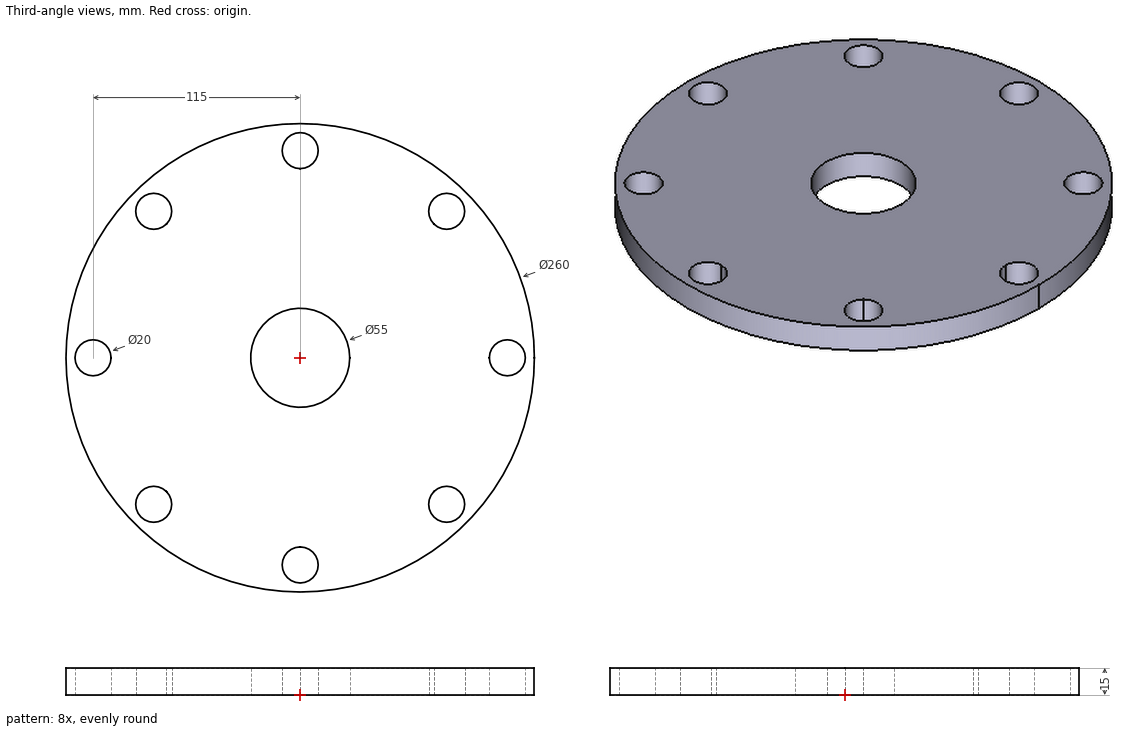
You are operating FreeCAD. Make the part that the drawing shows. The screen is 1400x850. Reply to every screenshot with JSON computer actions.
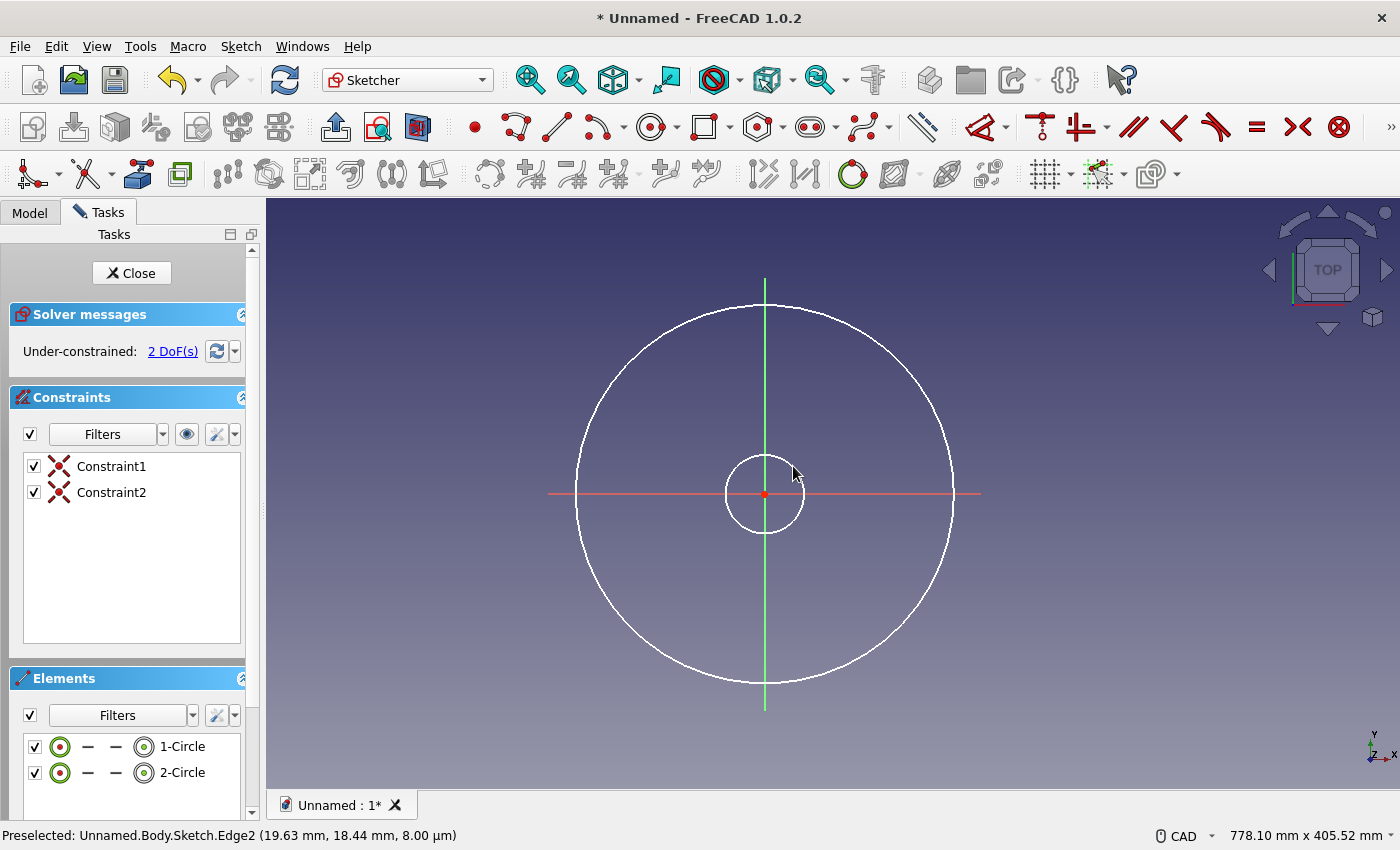
{"action": "left_click", "coordinate": [980, 128]}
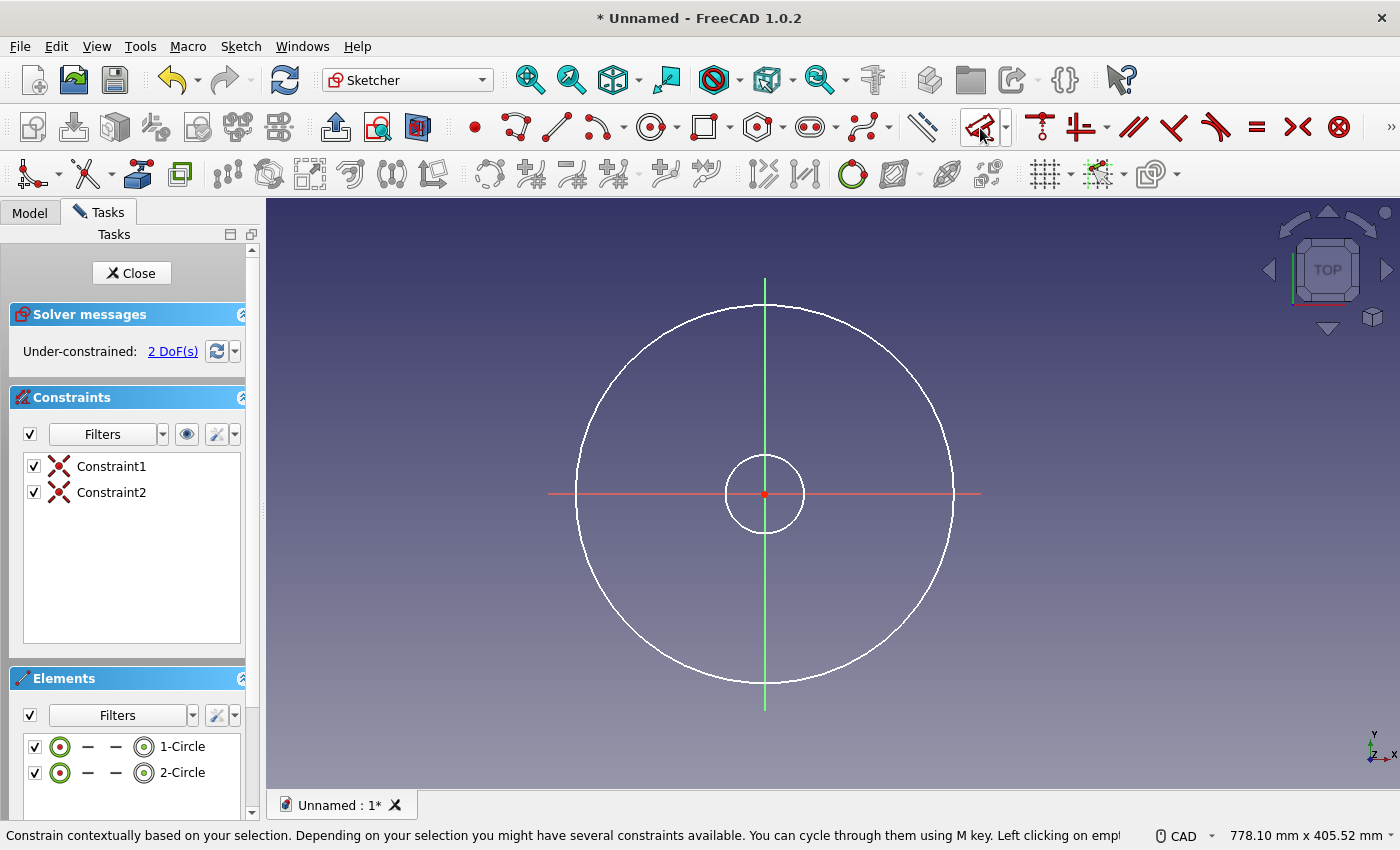
{"action": "left_click", "coordinate": [898, 360]}
{"action": "left_click", "coordinate": [921, 337]}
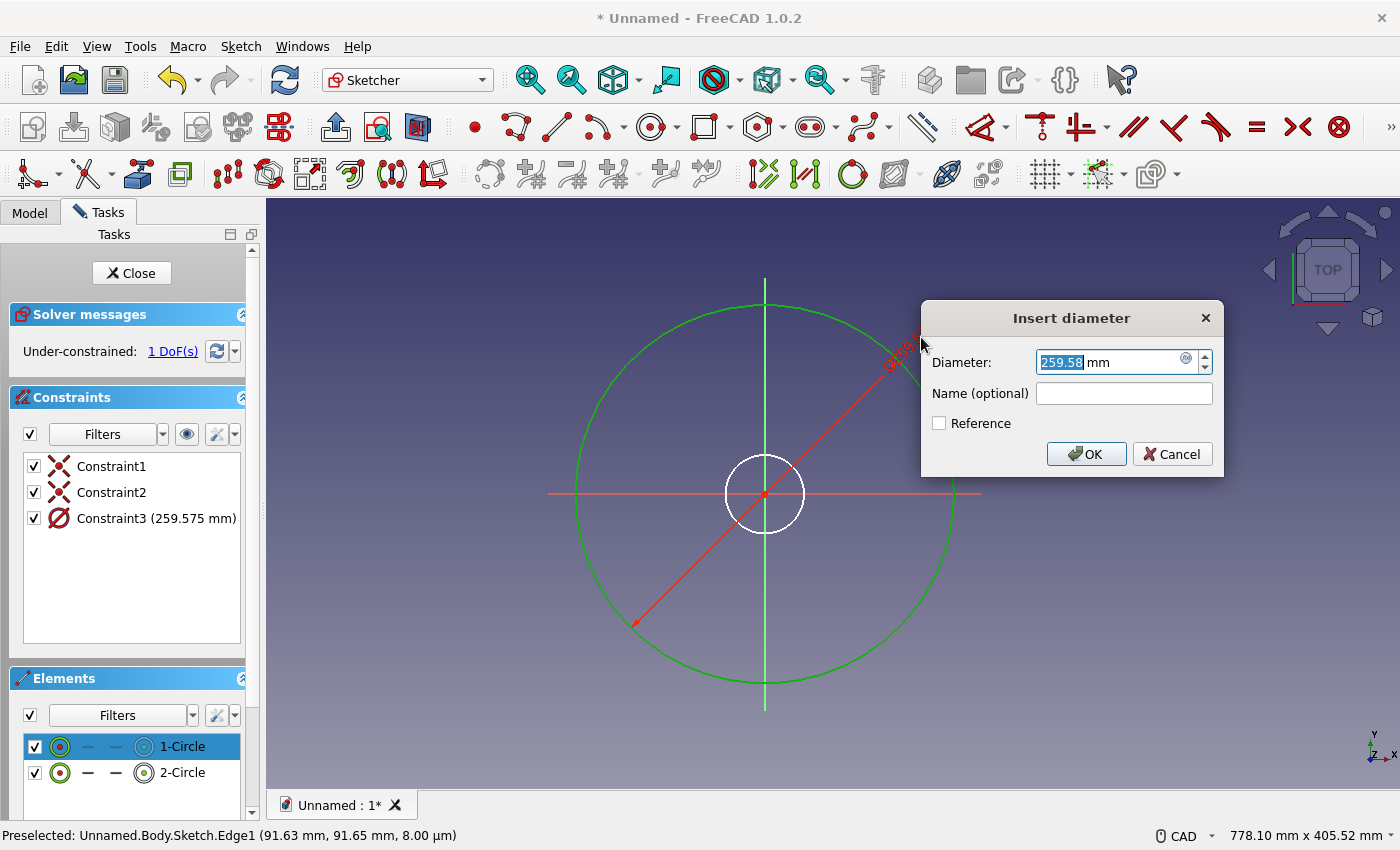
{"action": "type", "text": "260"}
{"action": "key", "text": "Return"}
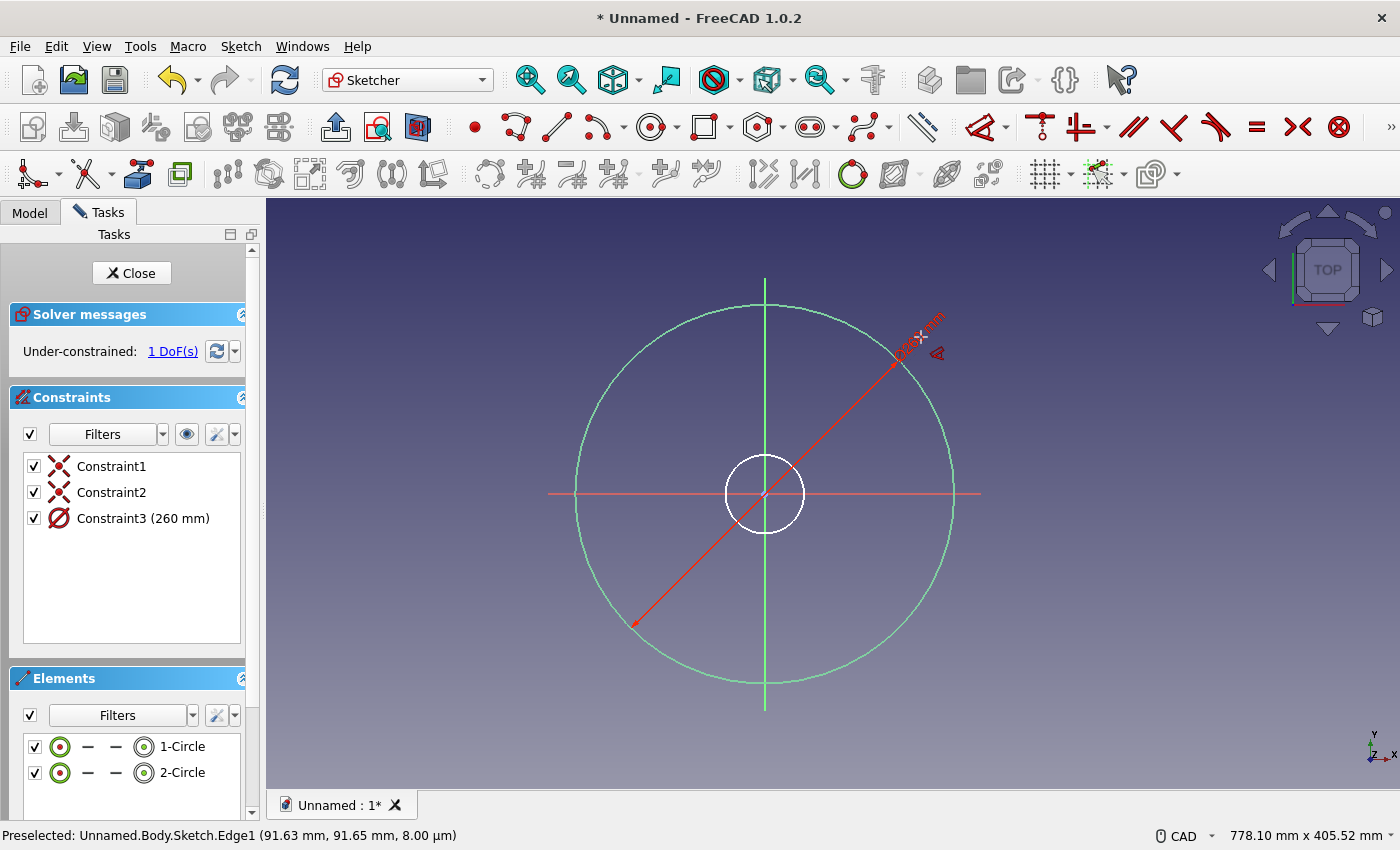
{"action": "left_click", "coordinate": [792, 466]}
{"action": "left_click", "coordinate": [814, 443]}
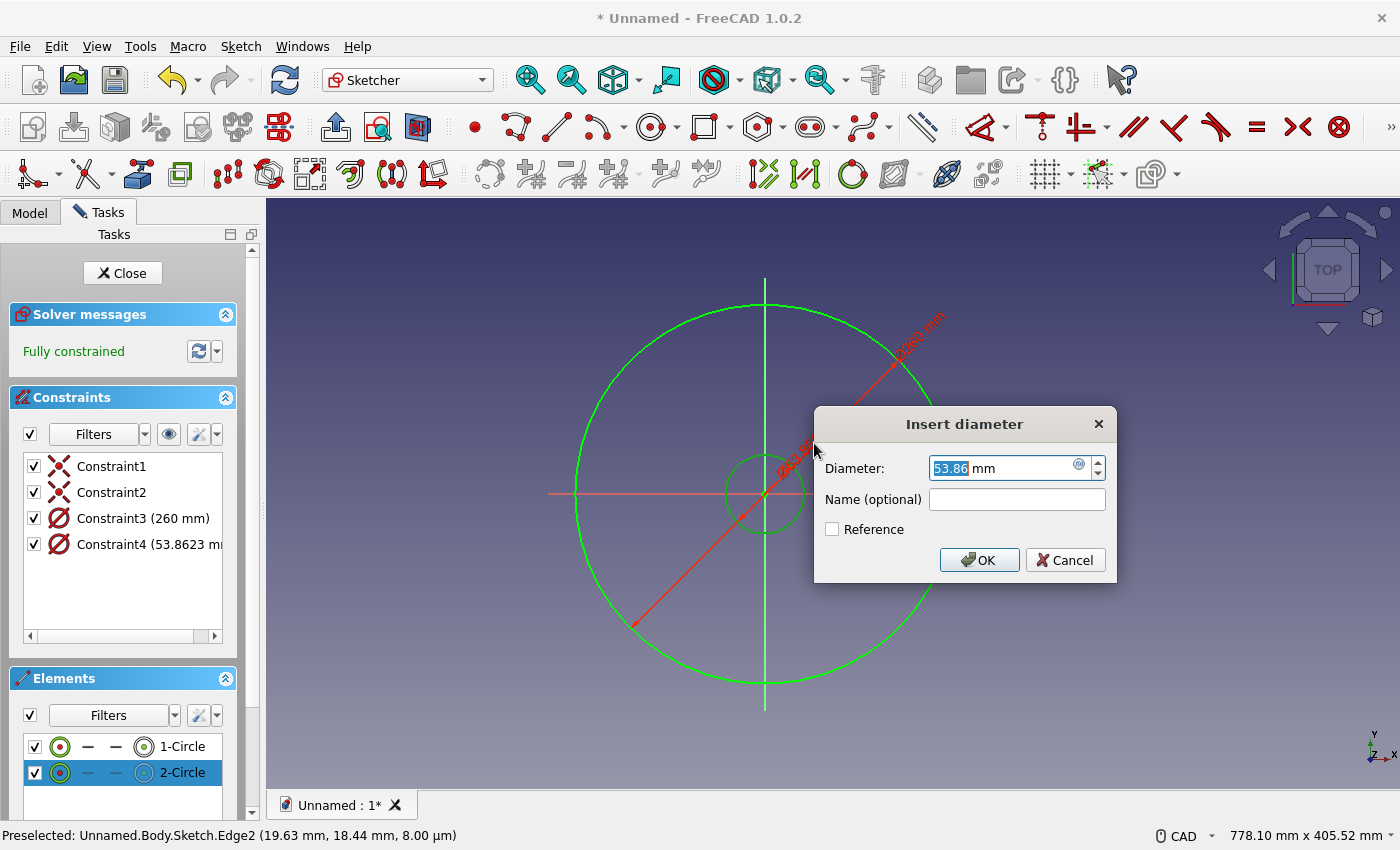
{"action": "type", "text": "55"}
{"action": "key", "text": "Return"}
{"action": "key", "text": "Escape"}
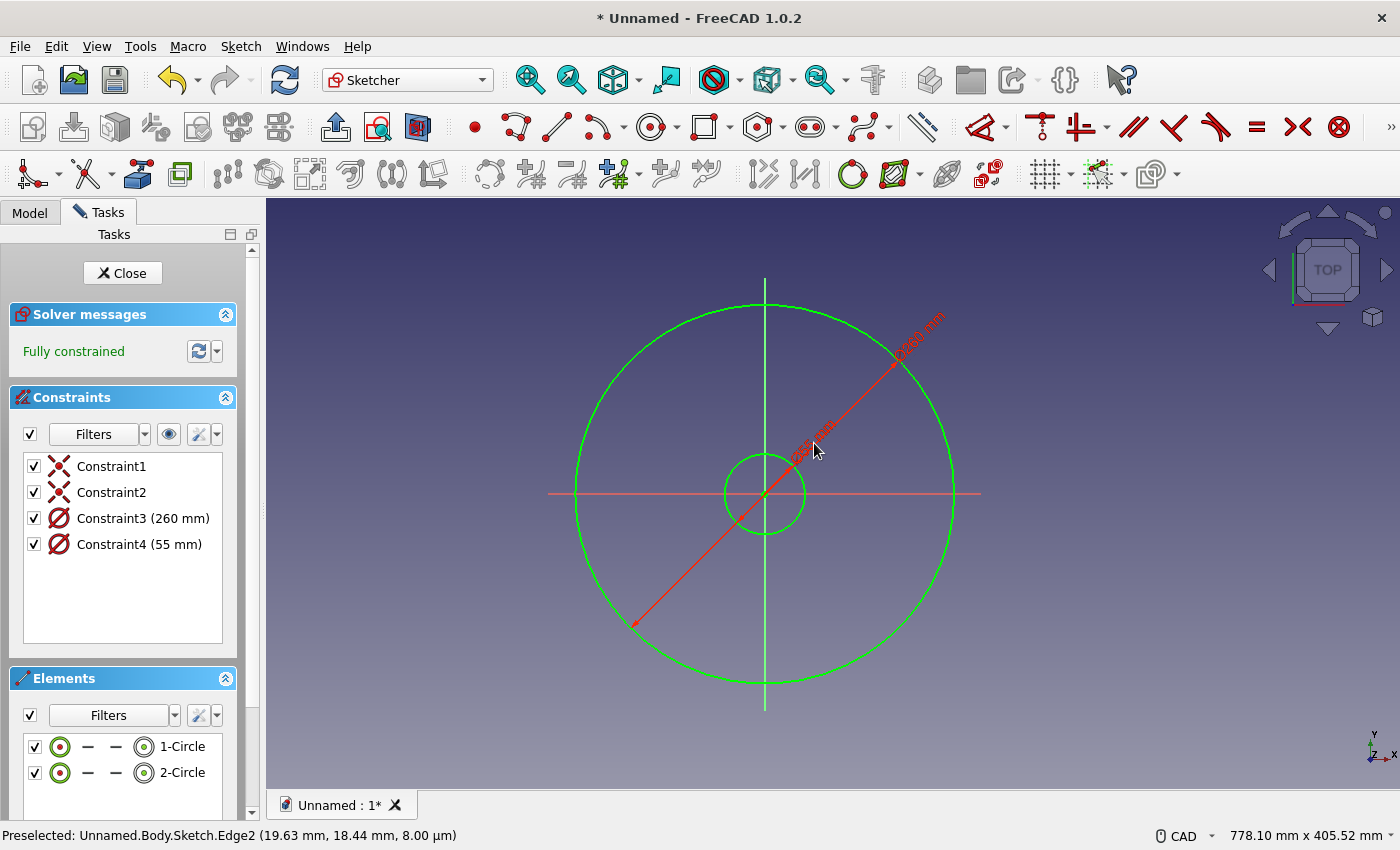
{"action": "left_click", "coordinate": [123, 273]}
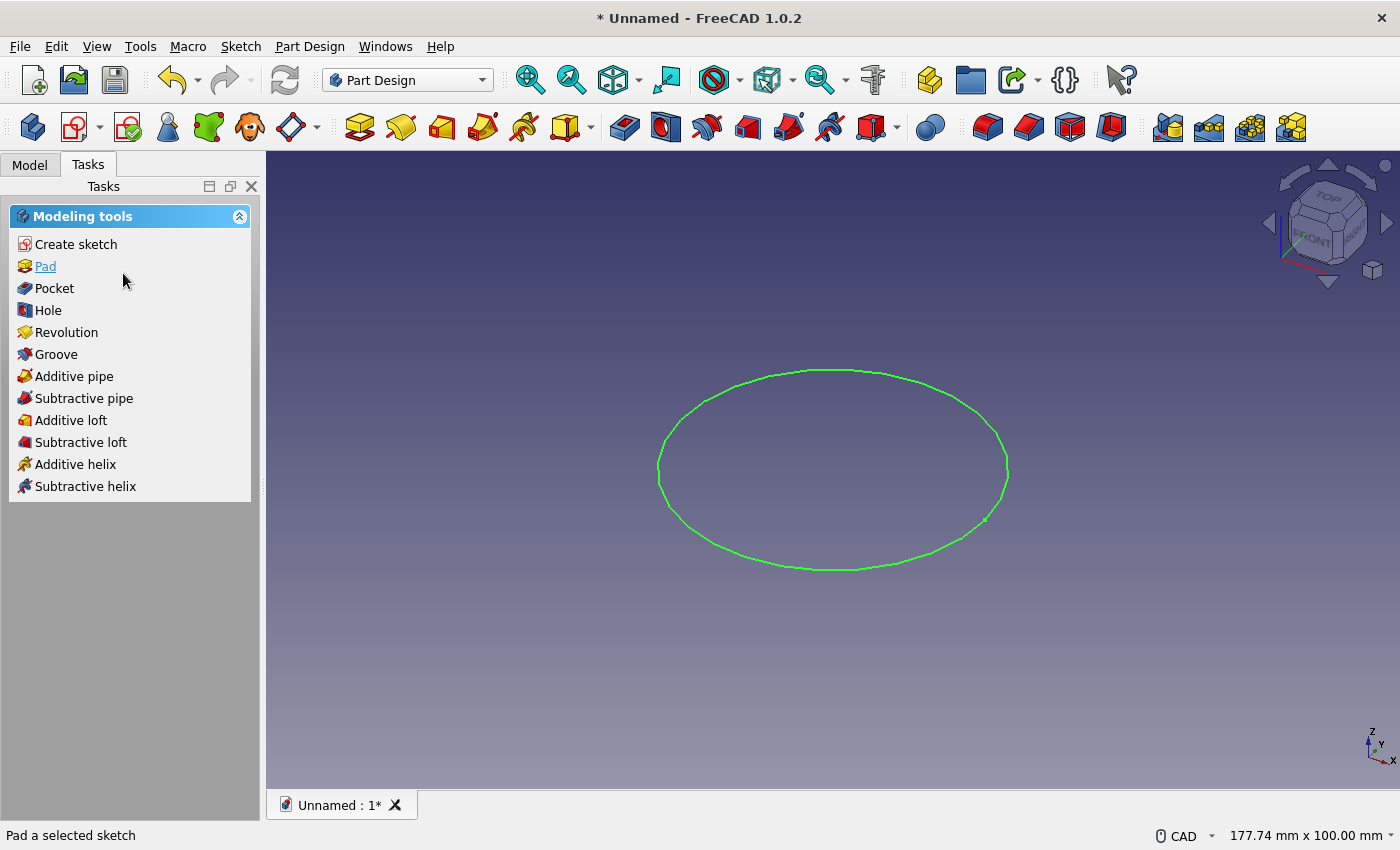
{"action": "left_click", "coordinate": [360, 128]}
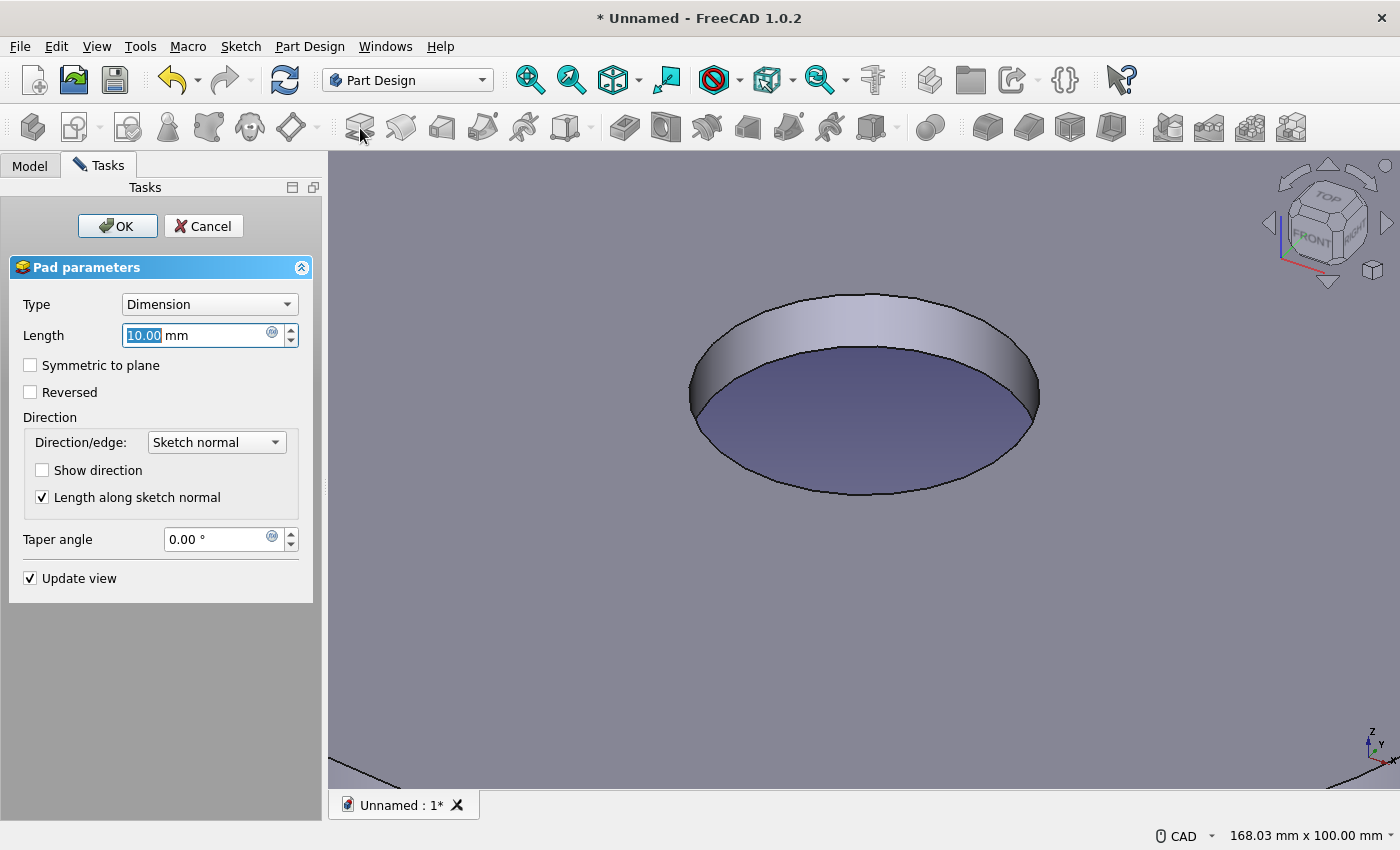
{"action": "type", "text": "15"}
{"action": "key", "text": "Tab"}